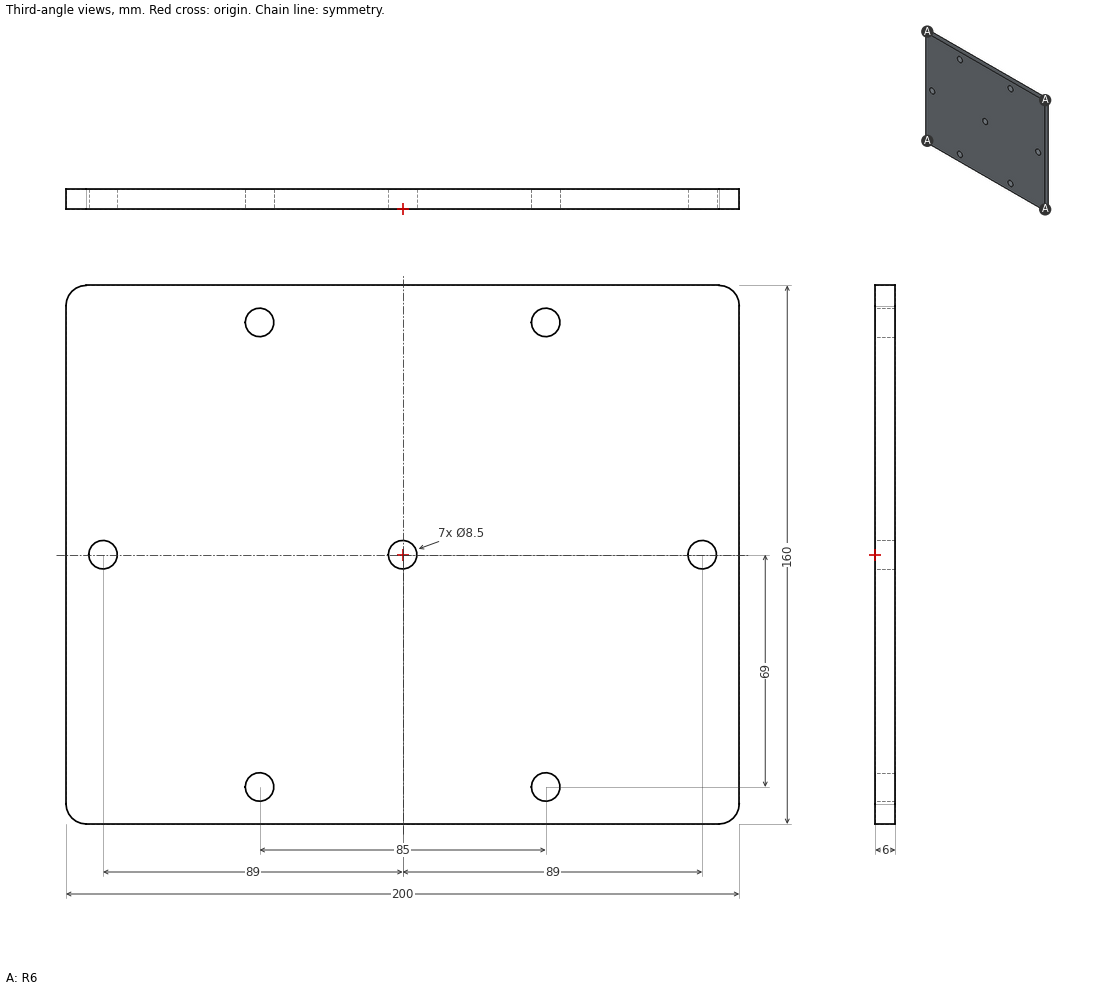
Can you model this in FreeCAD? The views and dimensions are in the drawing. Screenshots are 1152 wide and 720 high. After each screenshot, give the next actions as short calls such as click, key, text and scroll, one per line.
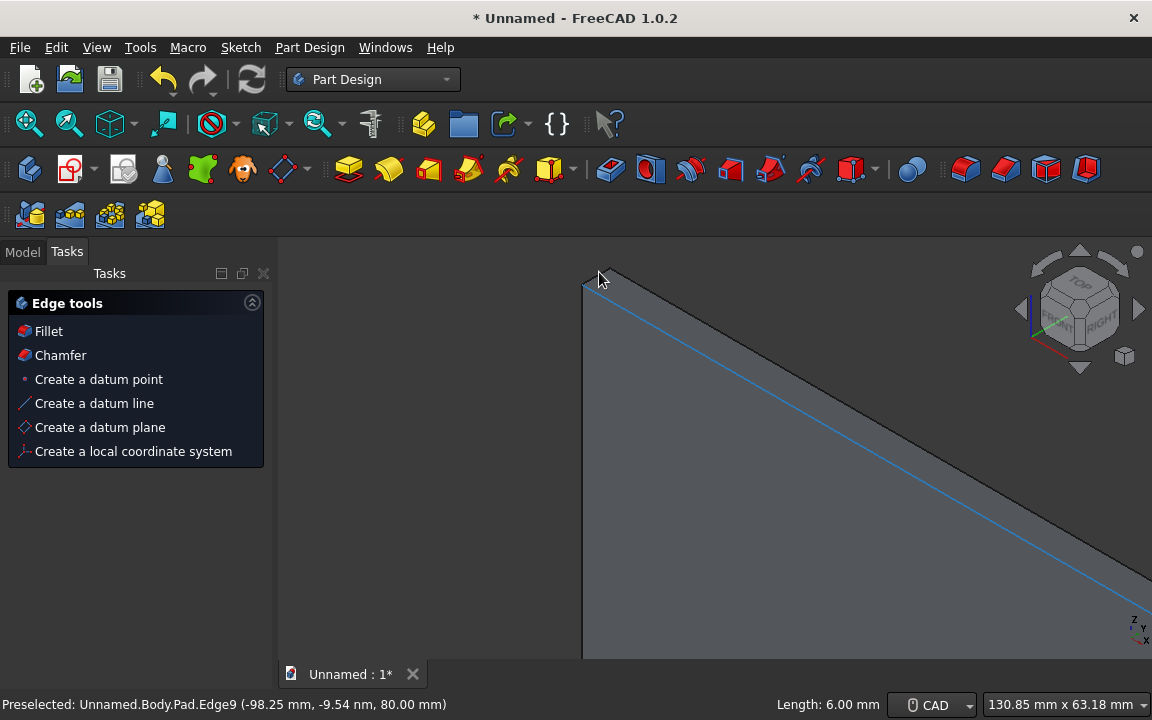
click(30, 124)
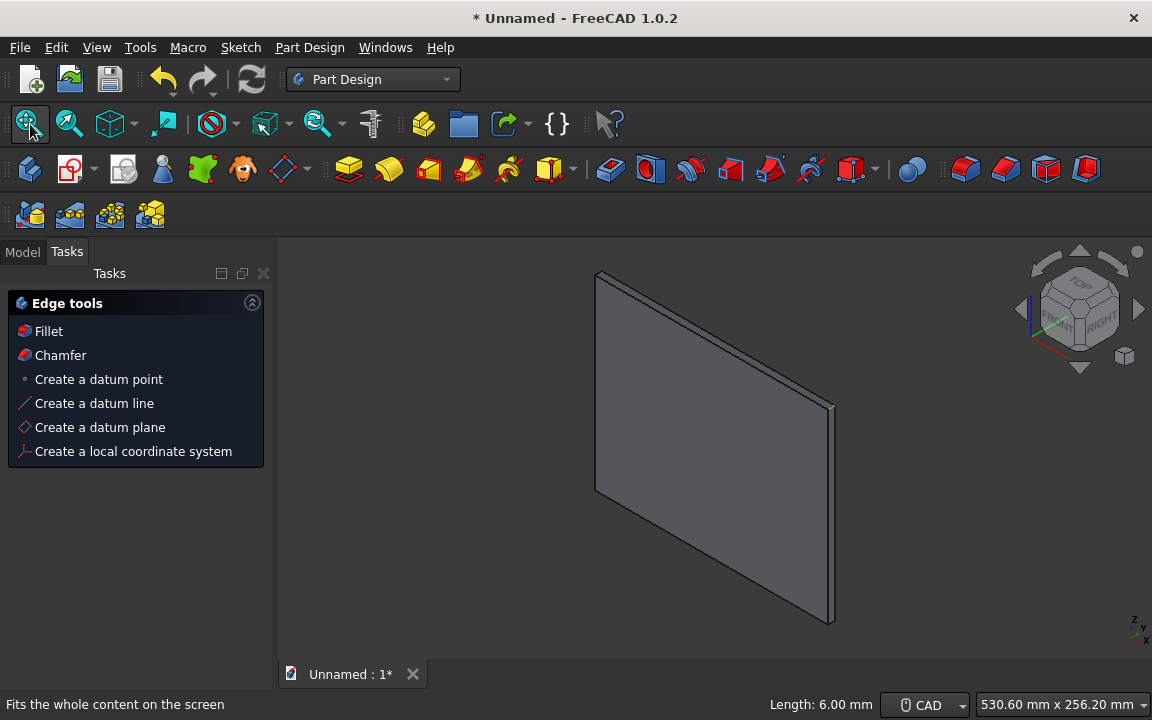
key(2)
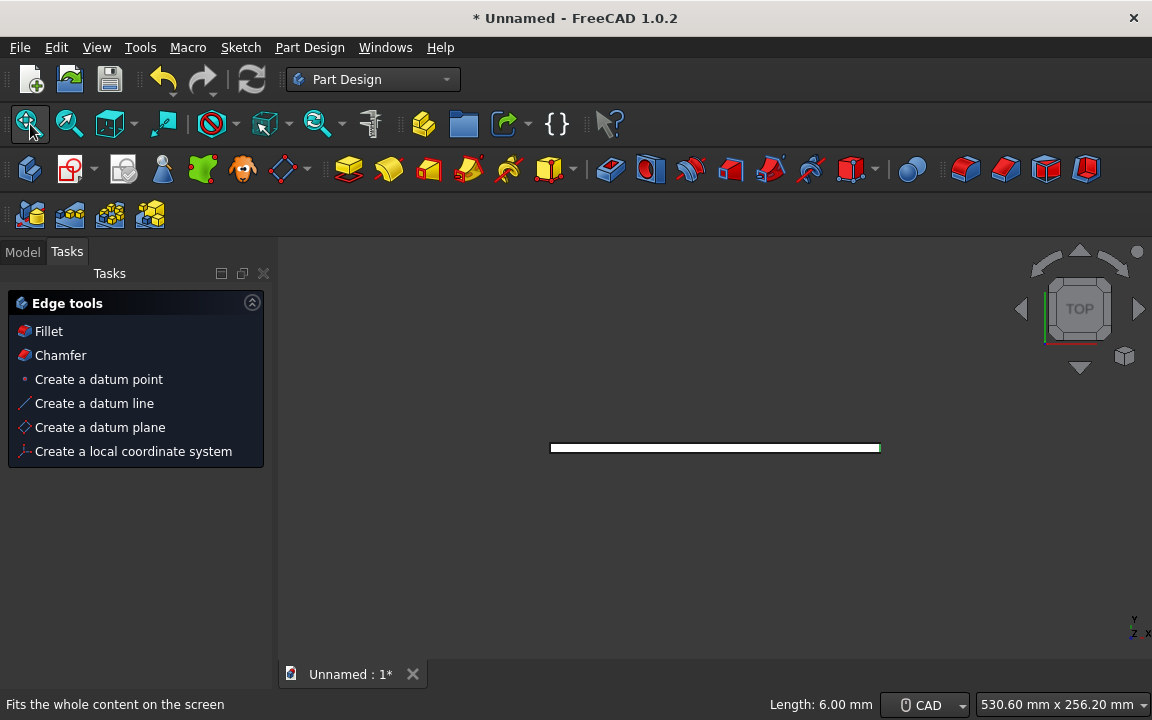
click(30, 124)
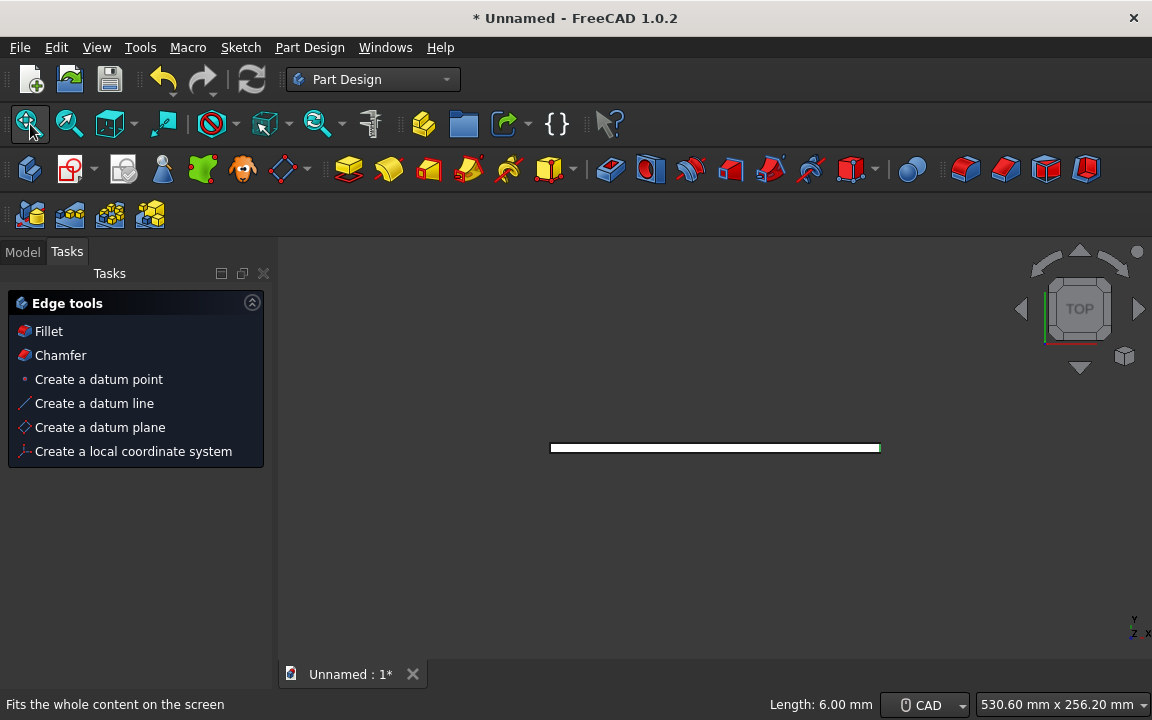
click(550, 449, ctrl)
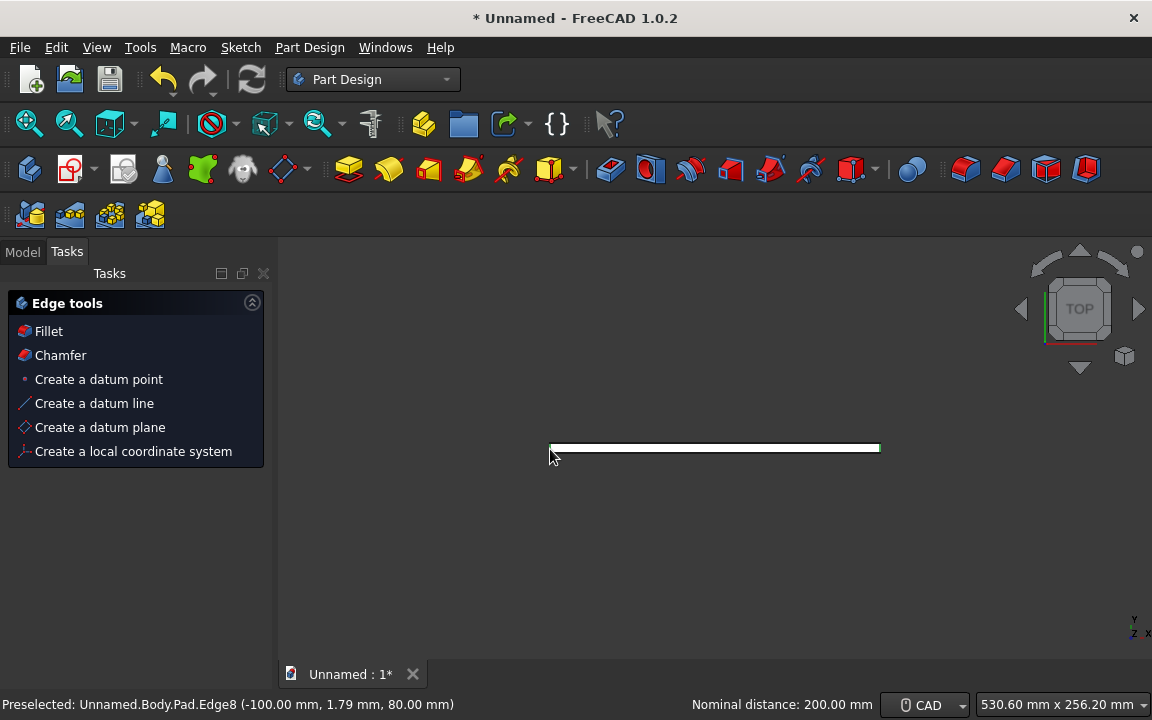
scroll(550, 447, up, 7)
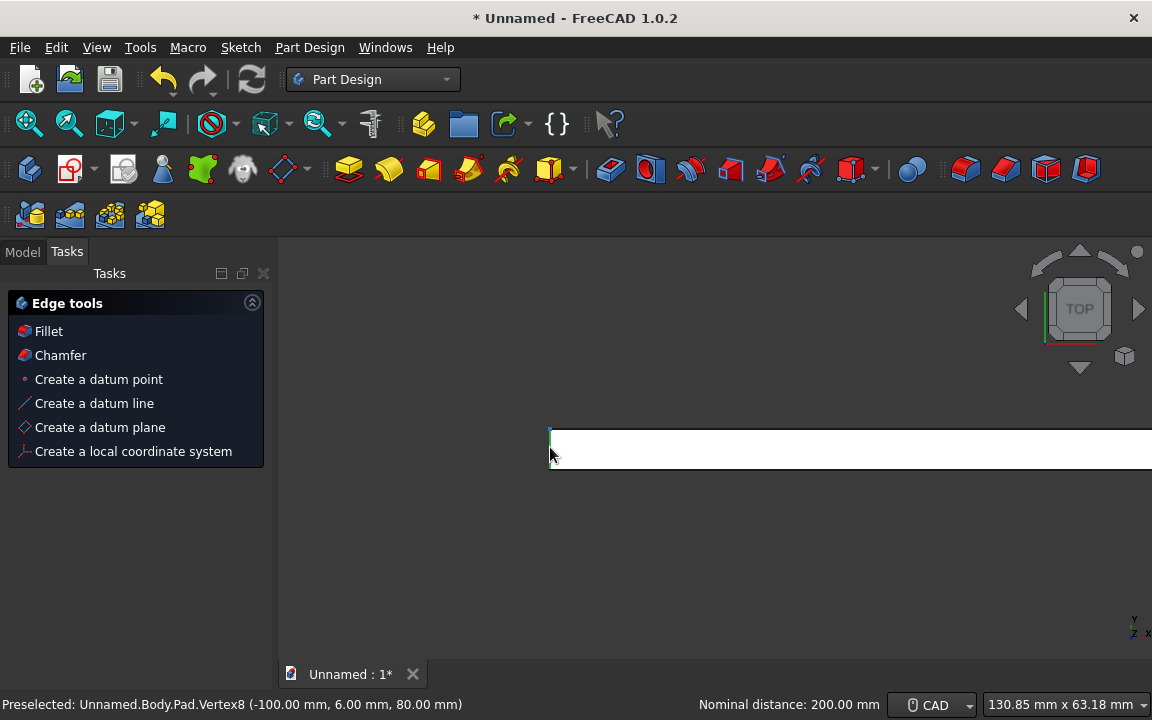
click(30, 124)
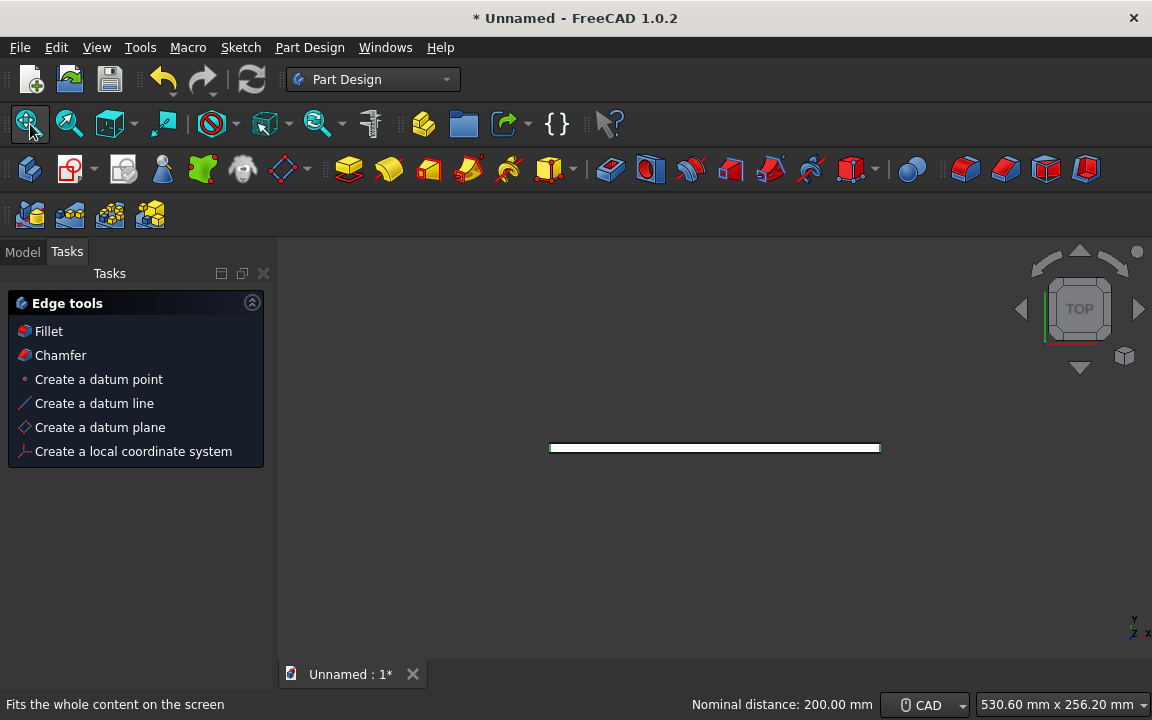
key(1)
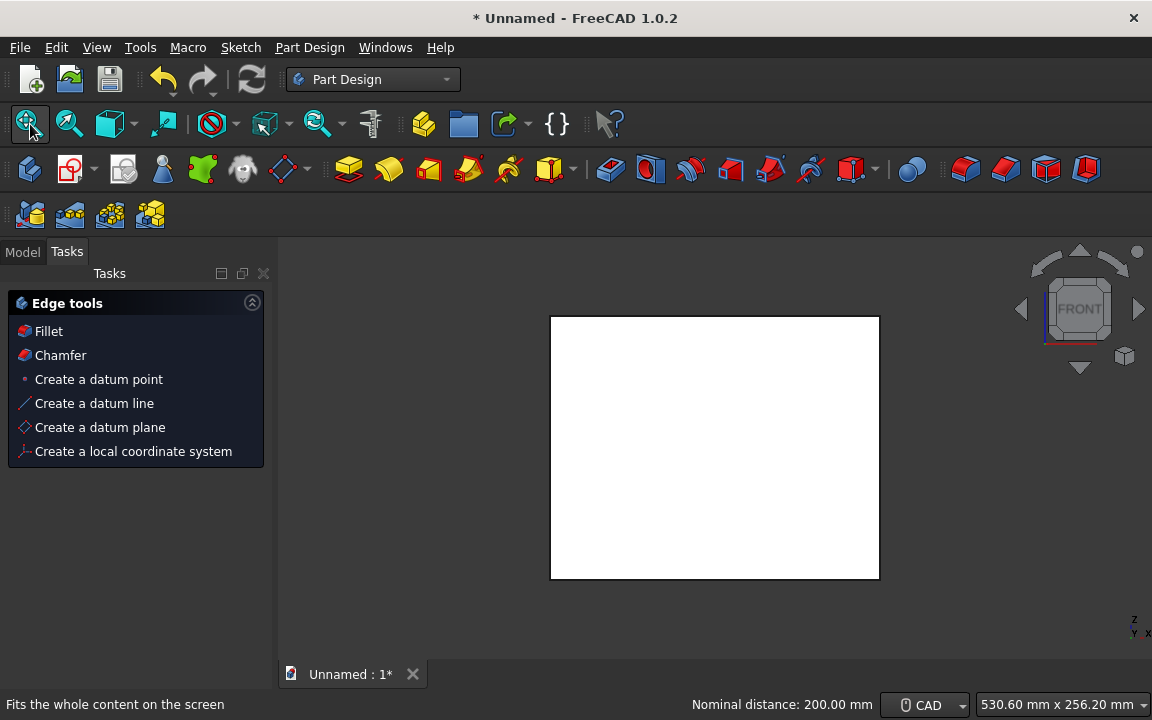
scroll(550, 579, up, 7)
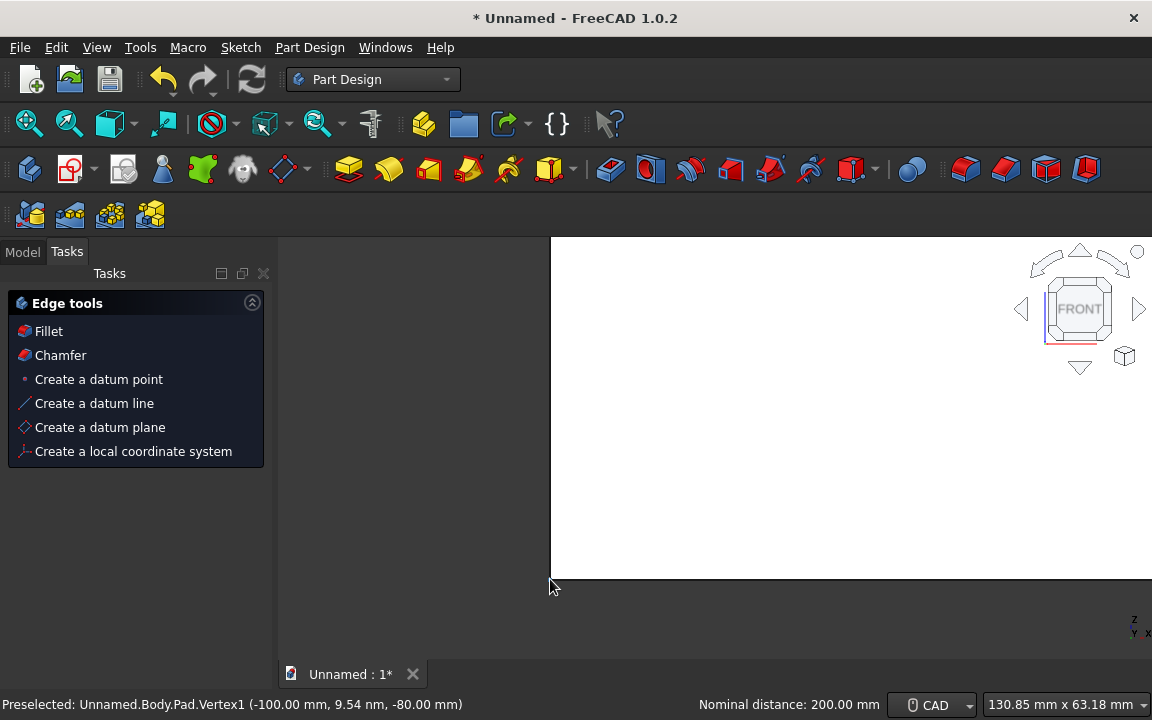
click(30, 124)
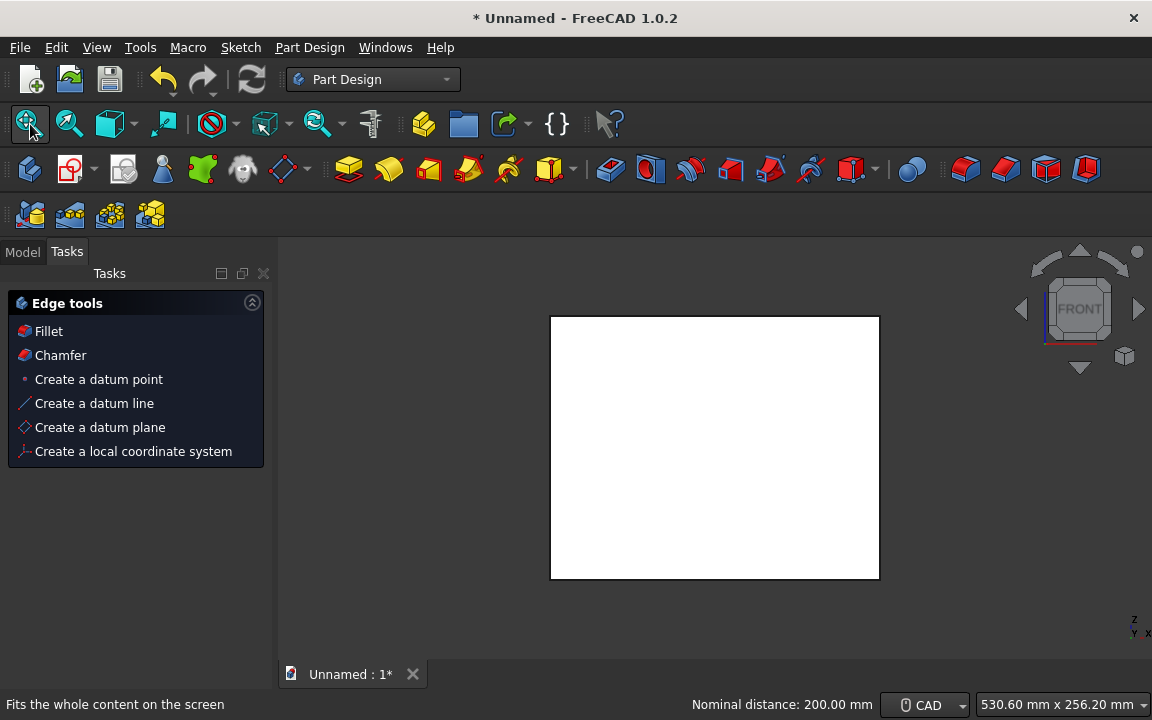
key(3)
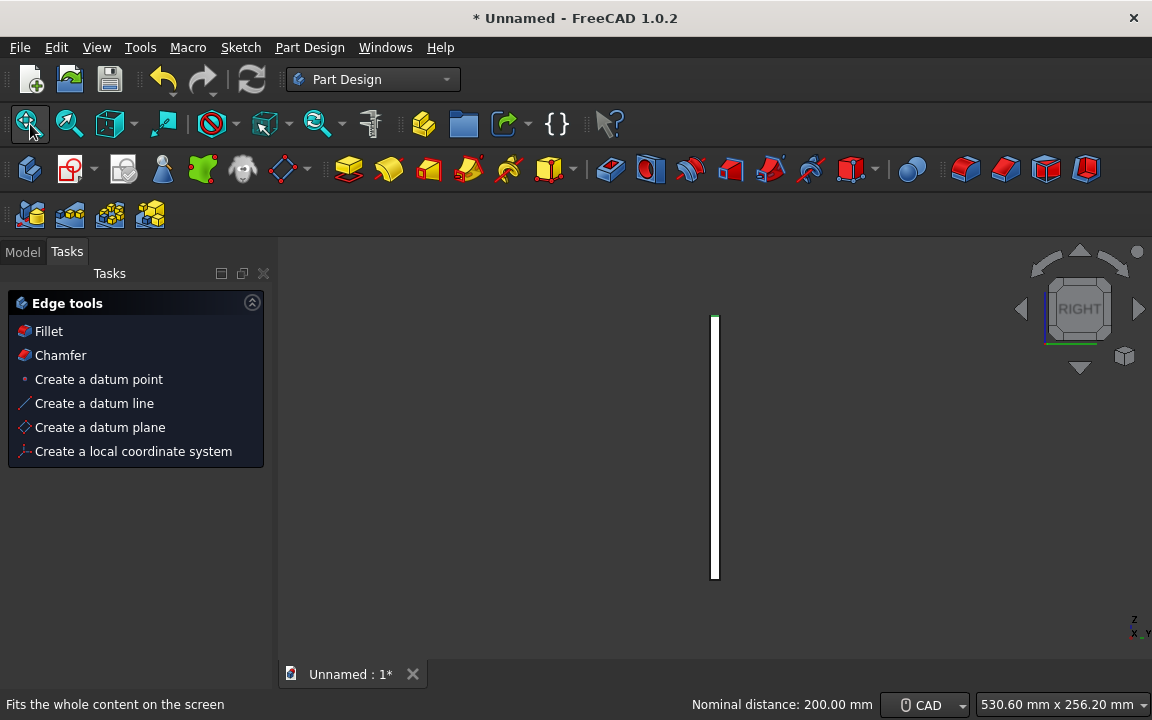
scroll(715, 579, up, 7)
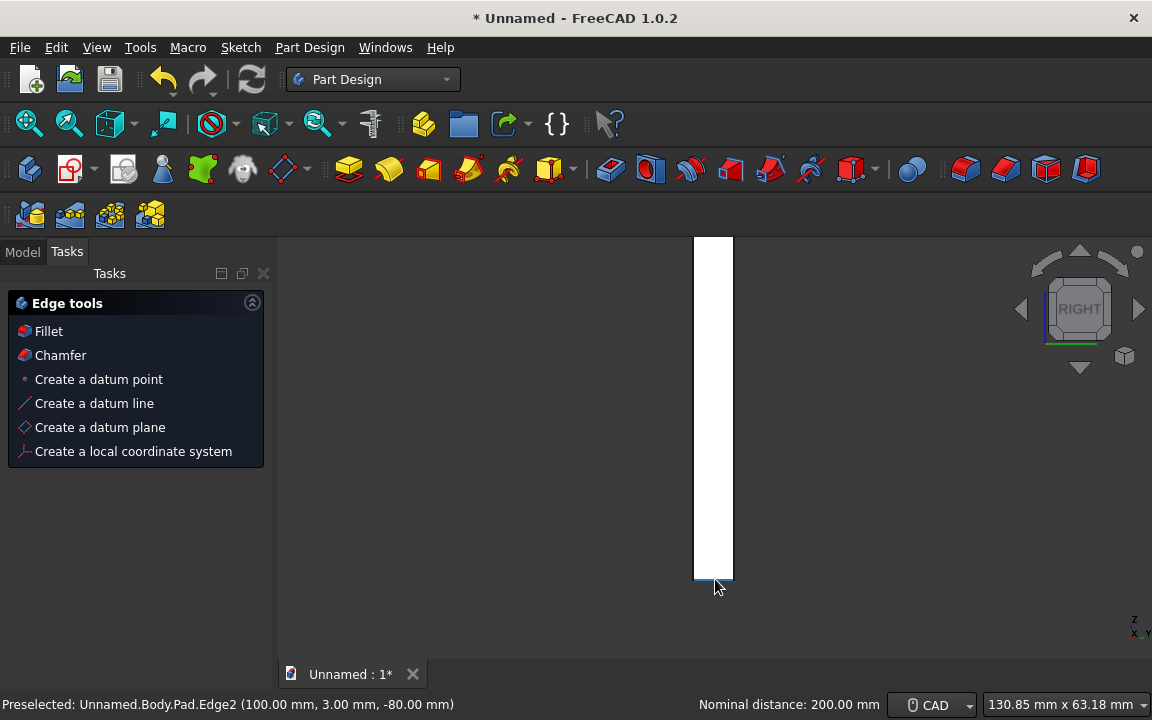
click(713, 579, ctrl)